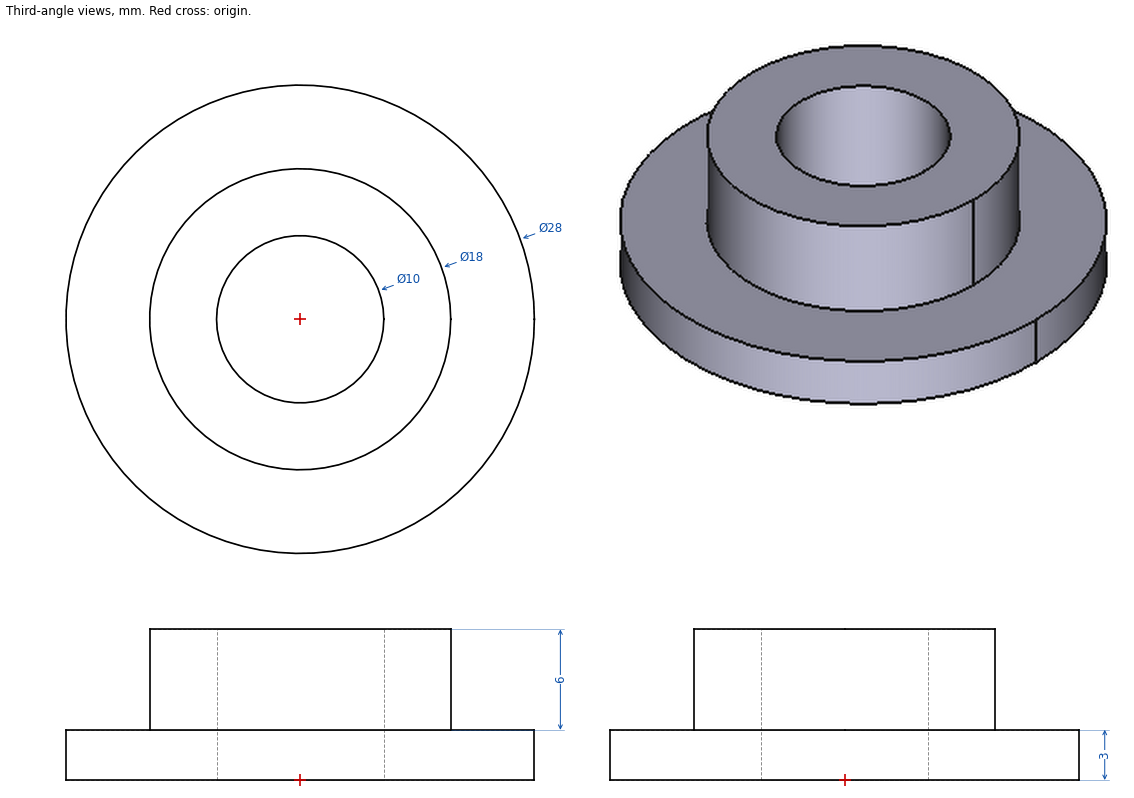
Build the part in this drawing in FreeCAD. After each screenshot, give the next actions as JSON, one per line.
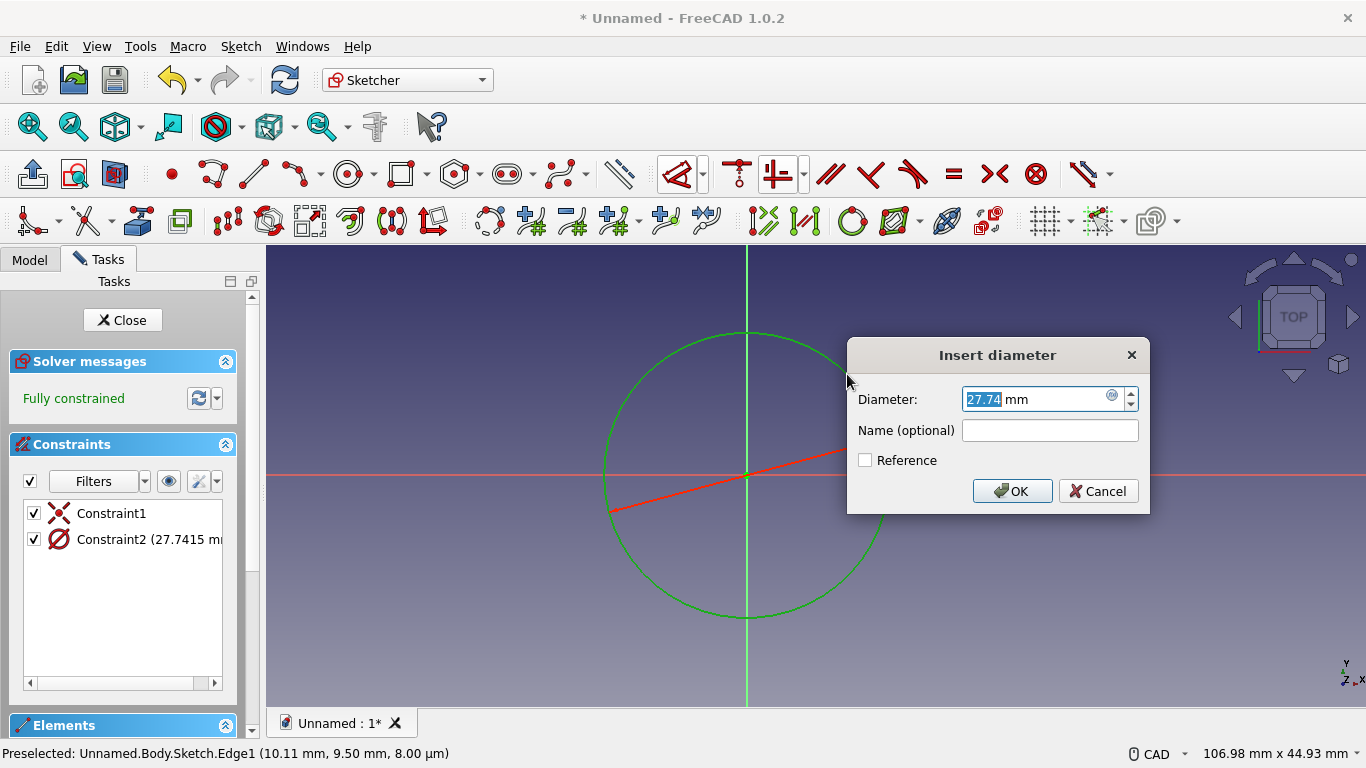
{"action": "type", "text": "28"}
{"action": "key", "text": "Return"}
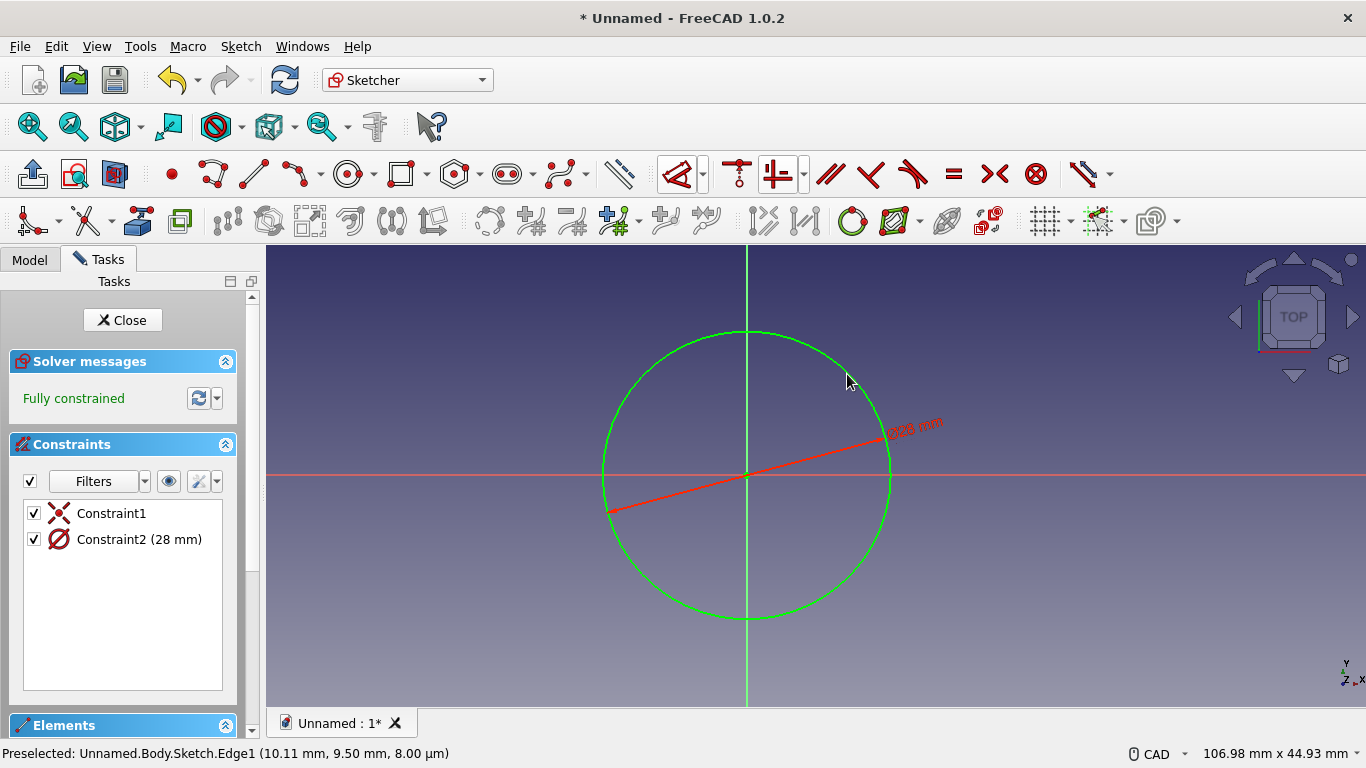
{"action": "left_click", "coordinate": [123, 320]}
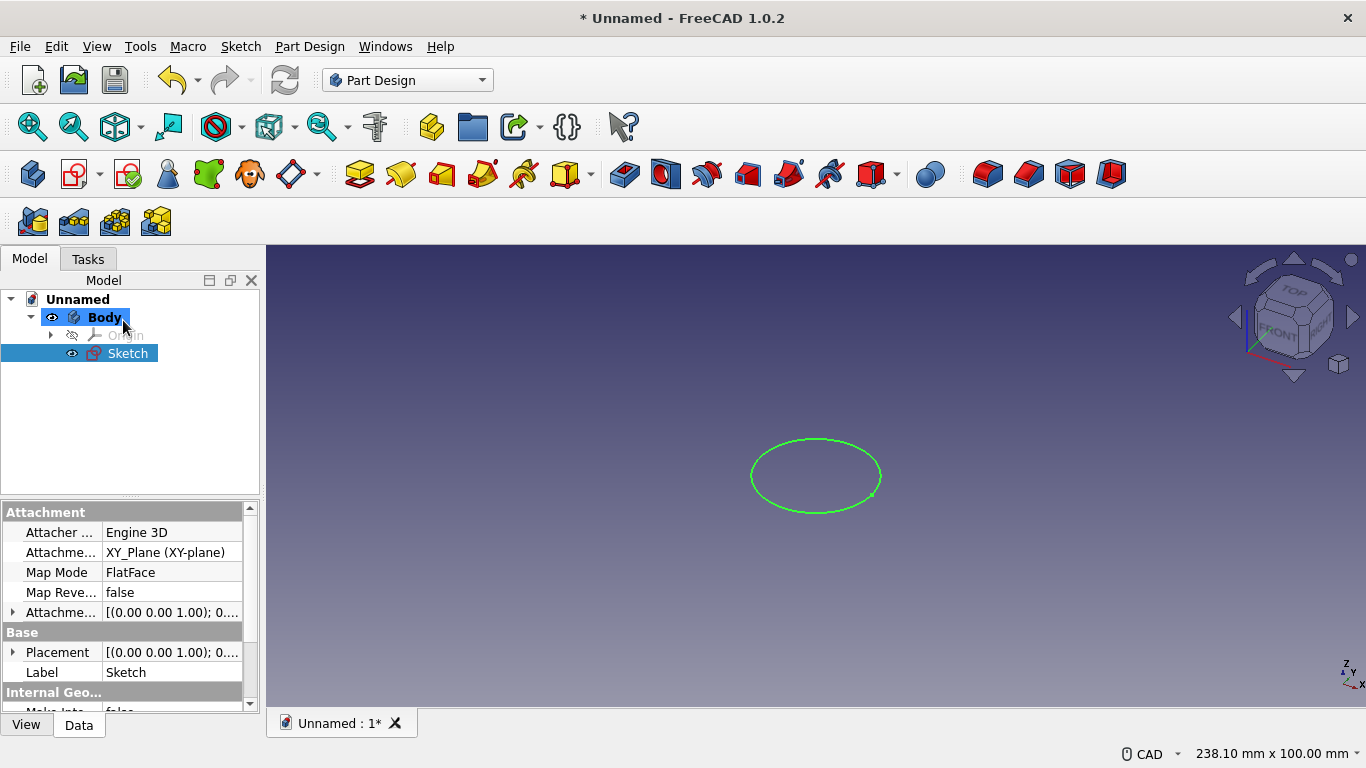
{"action": "left_click", "coordinate": [360, 174]}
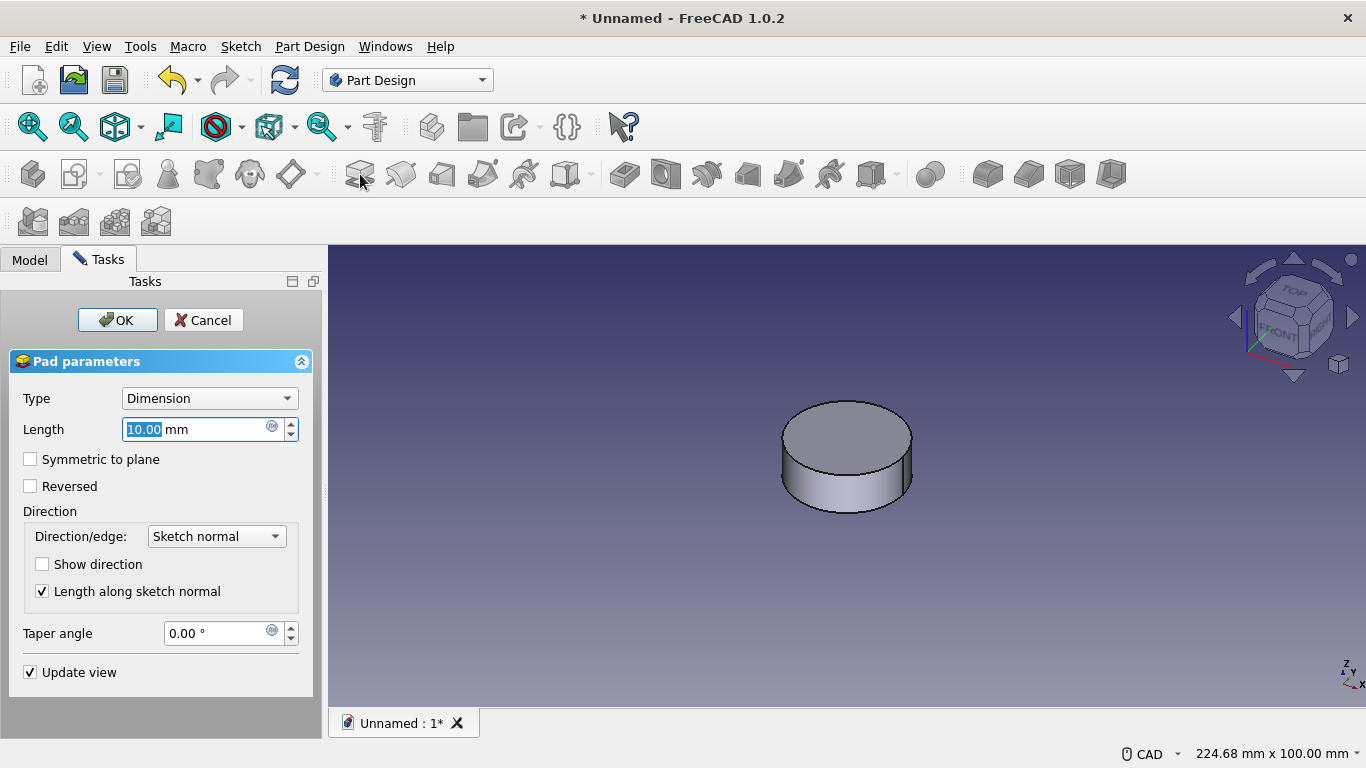
{"action": "type", "text": "3"}
{"action": "key", "text": "Tab"}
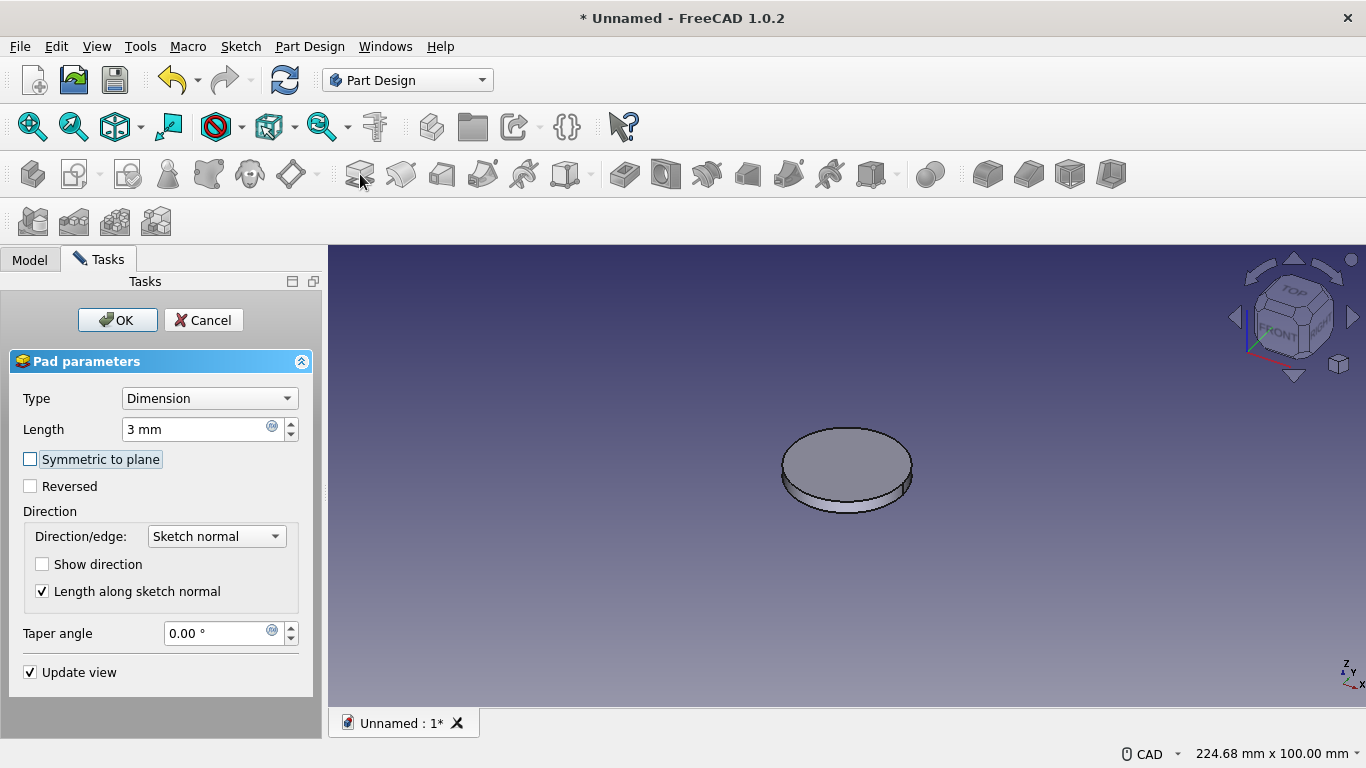
{"action": "left_click", "coordinate": [118, 320]}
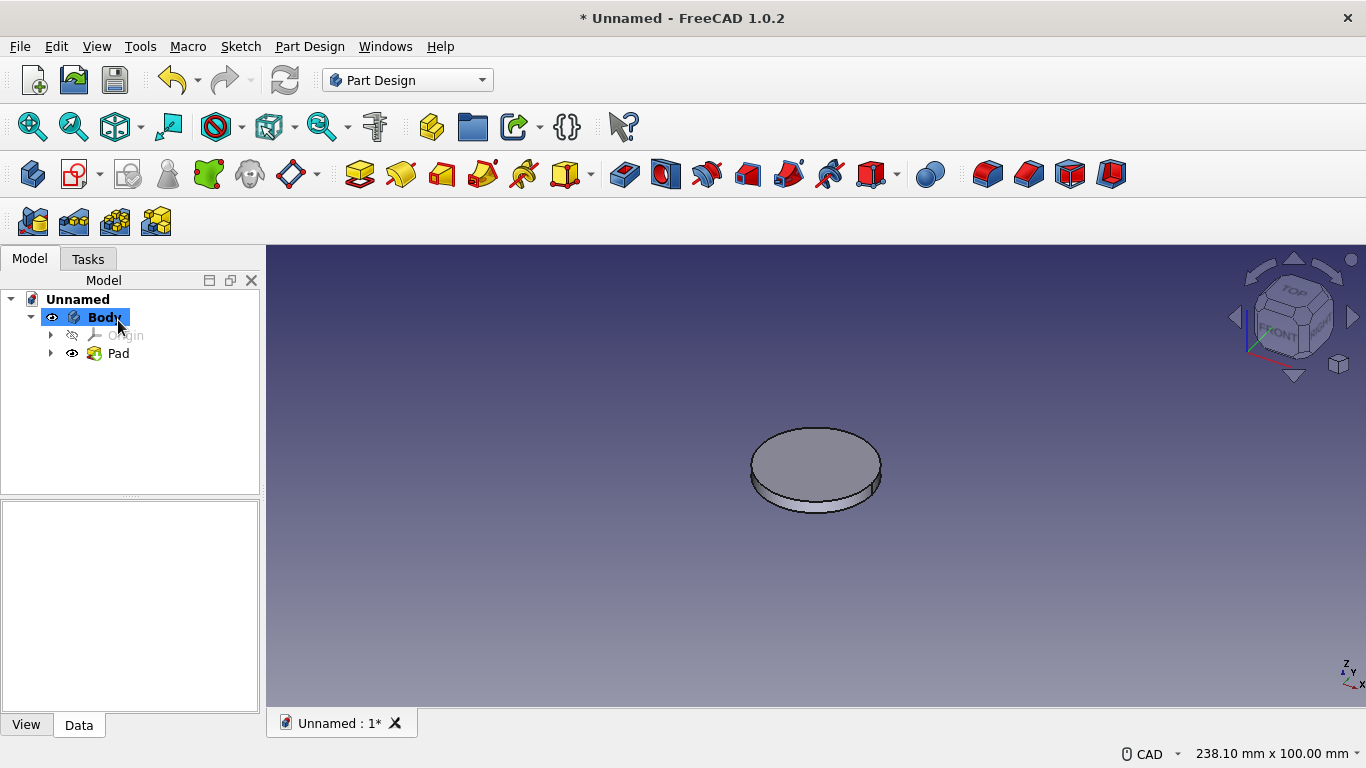
{"action": "key", "text": "v f"}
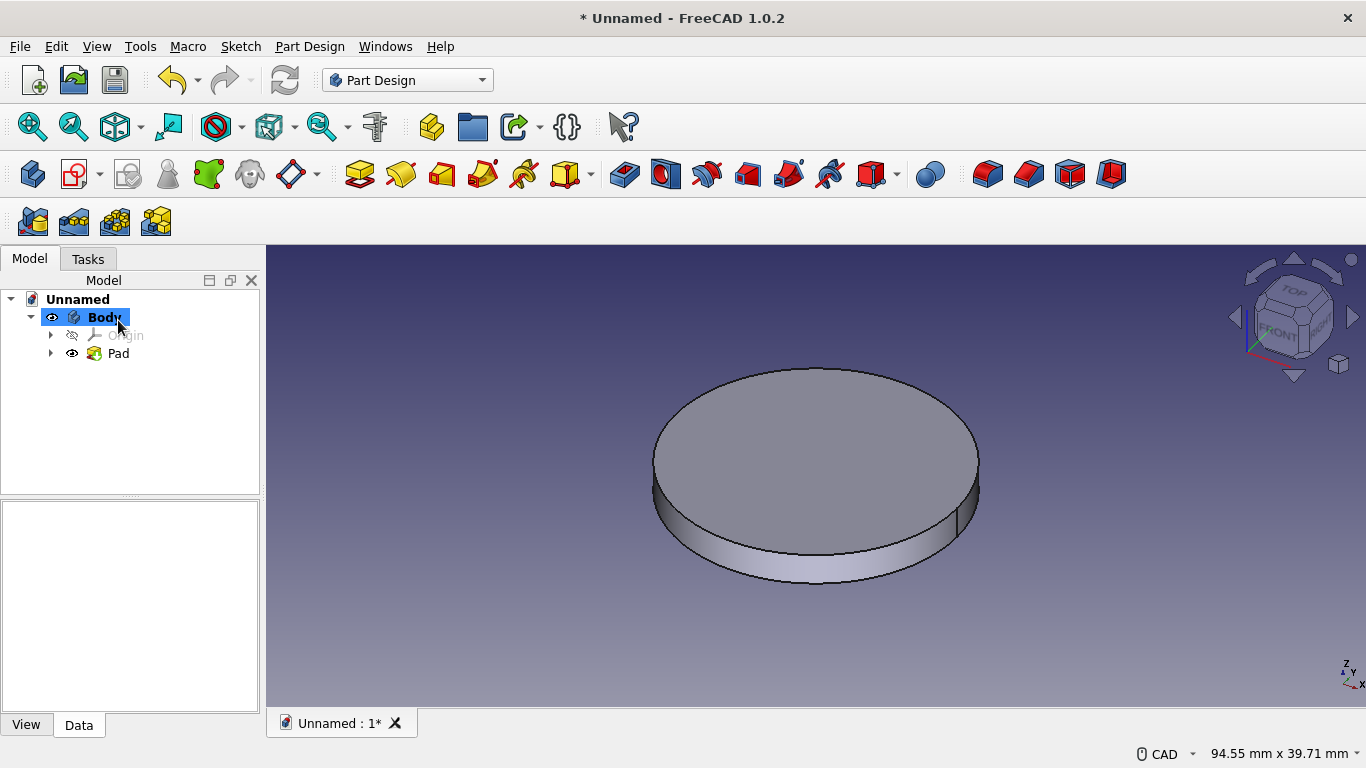
{"action": "left_click", "coordinate": [816, 461]}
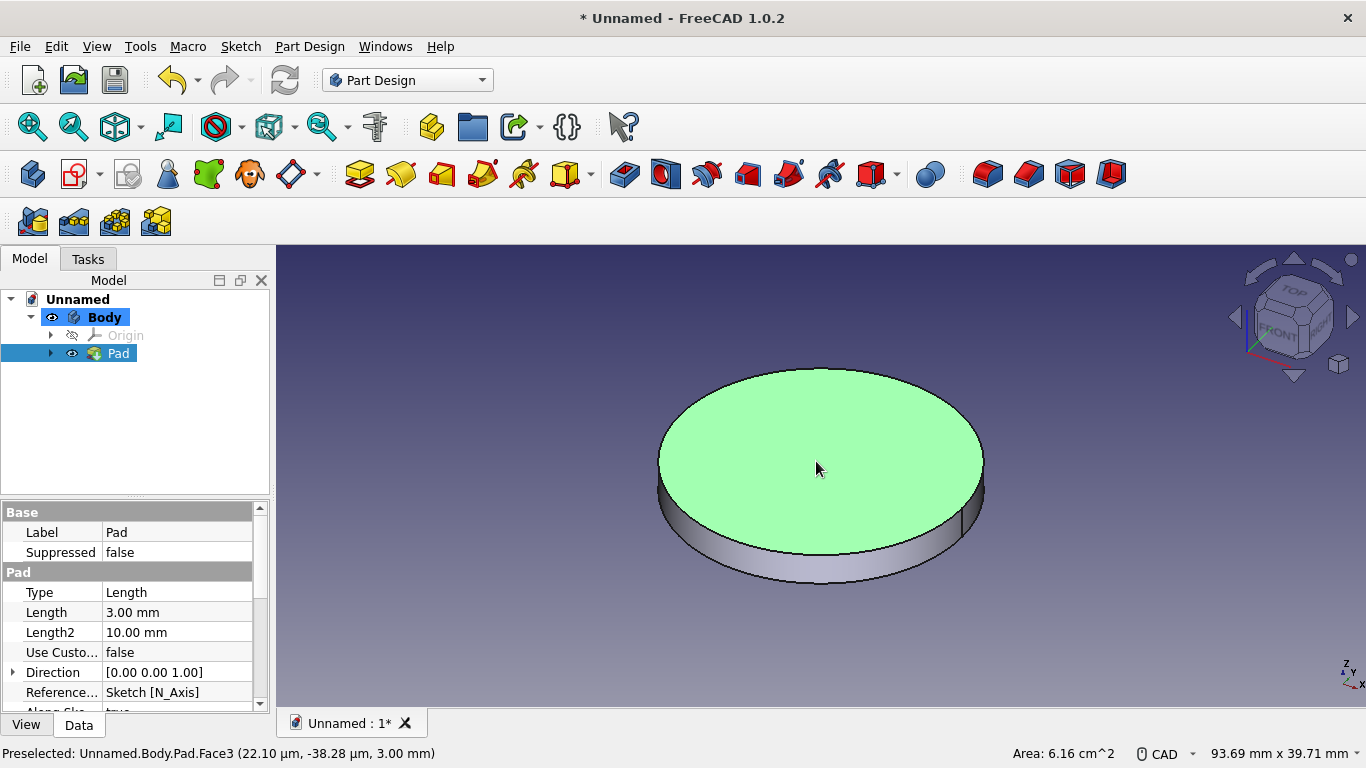
{"action": "left_click", "coordinate": [74, 174]}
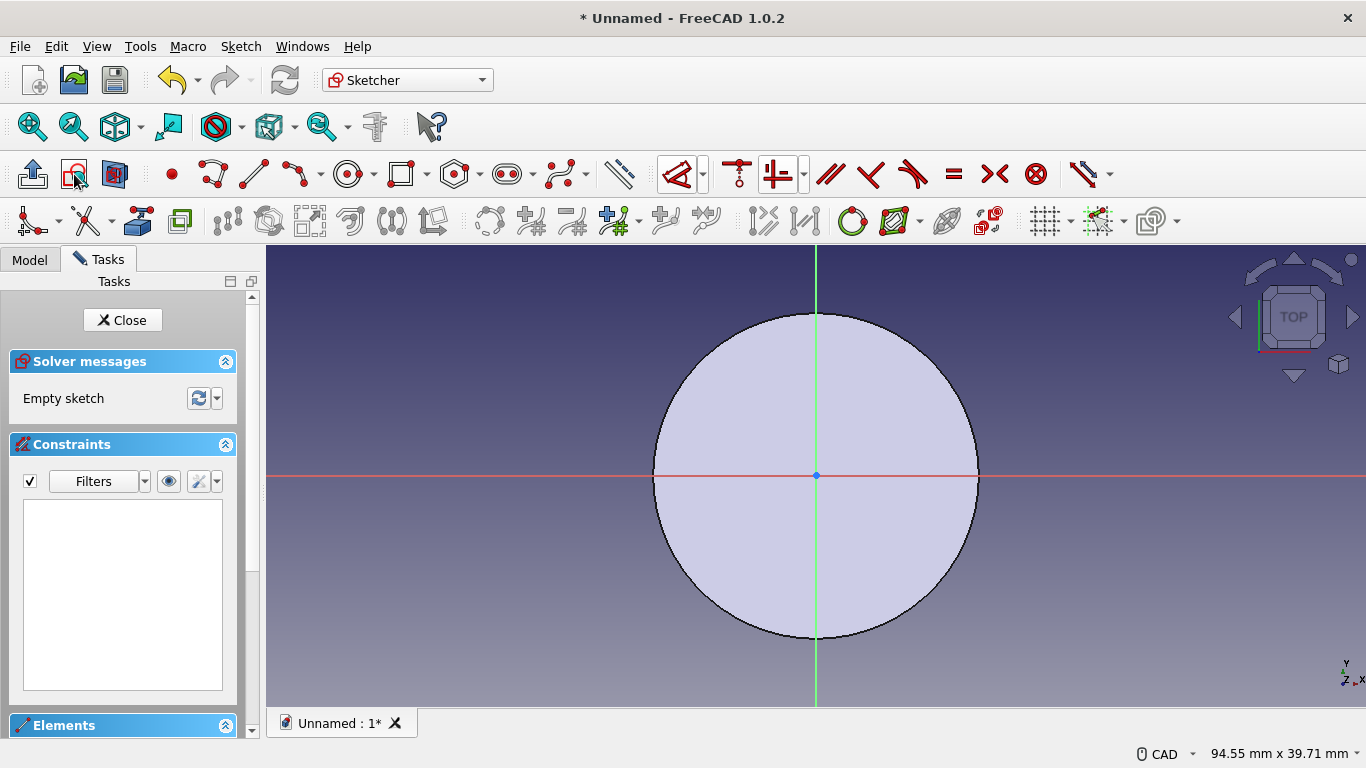
{"action": "scroll", "coordinate": [955, 476], "scroll_direction": "up", "scroll_amount": 2}